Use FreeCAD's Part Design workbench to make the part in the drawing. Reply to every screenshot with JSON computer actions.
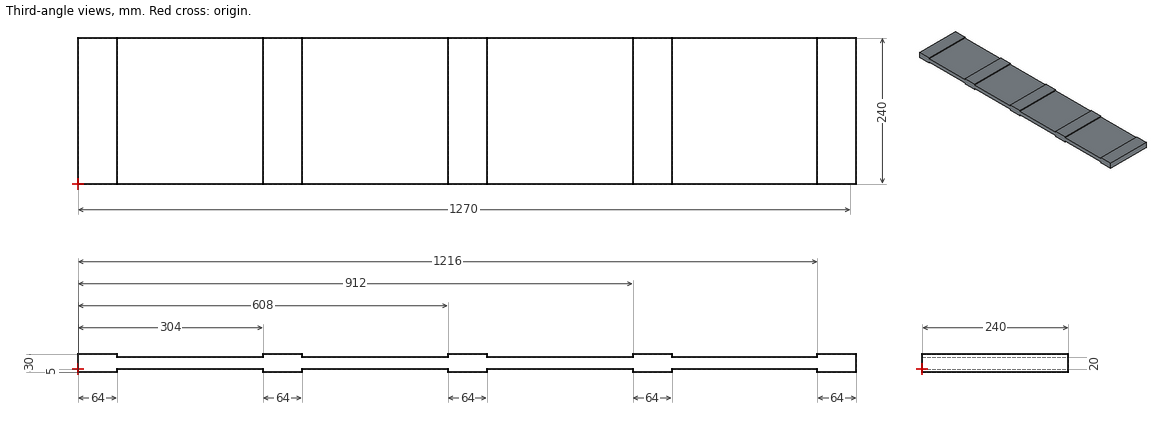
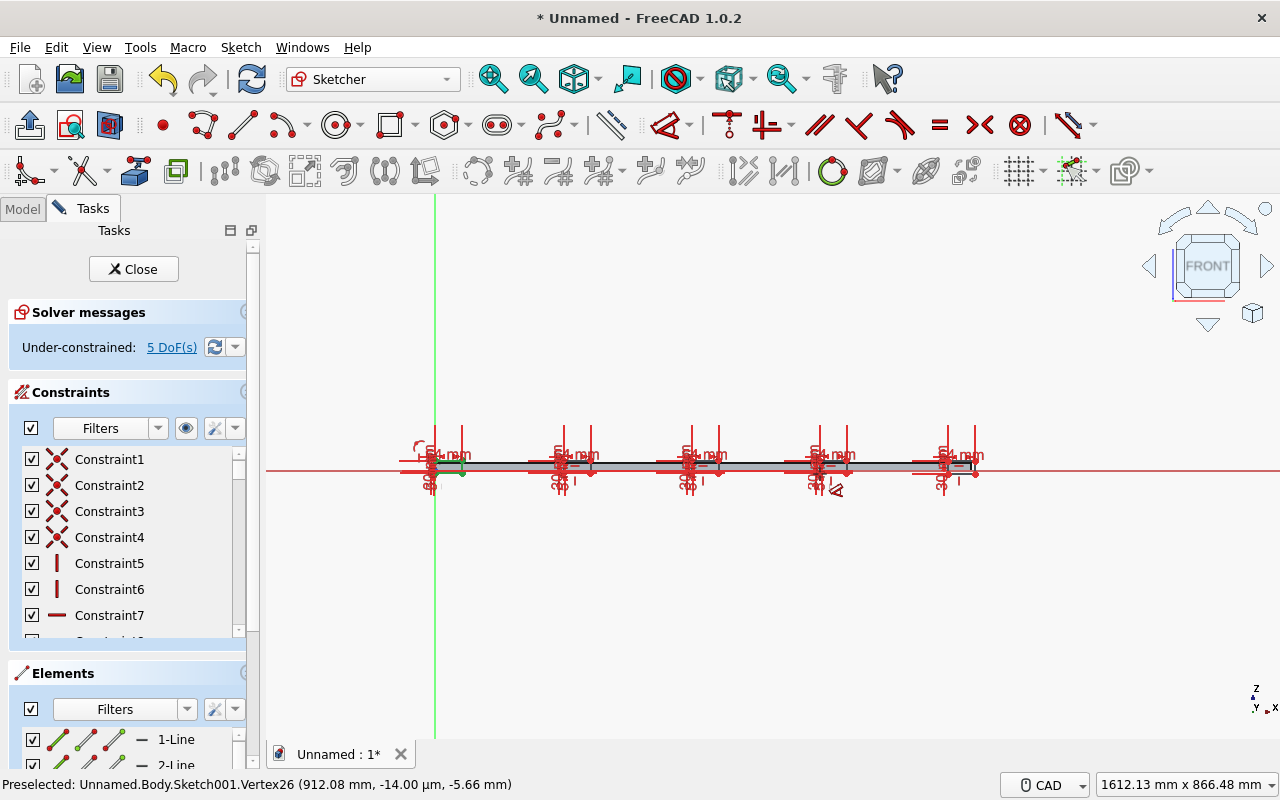
{"action": "scroll", "coordinate": [948, 474], "scroll_direction": "up", "scroll_amount": 15}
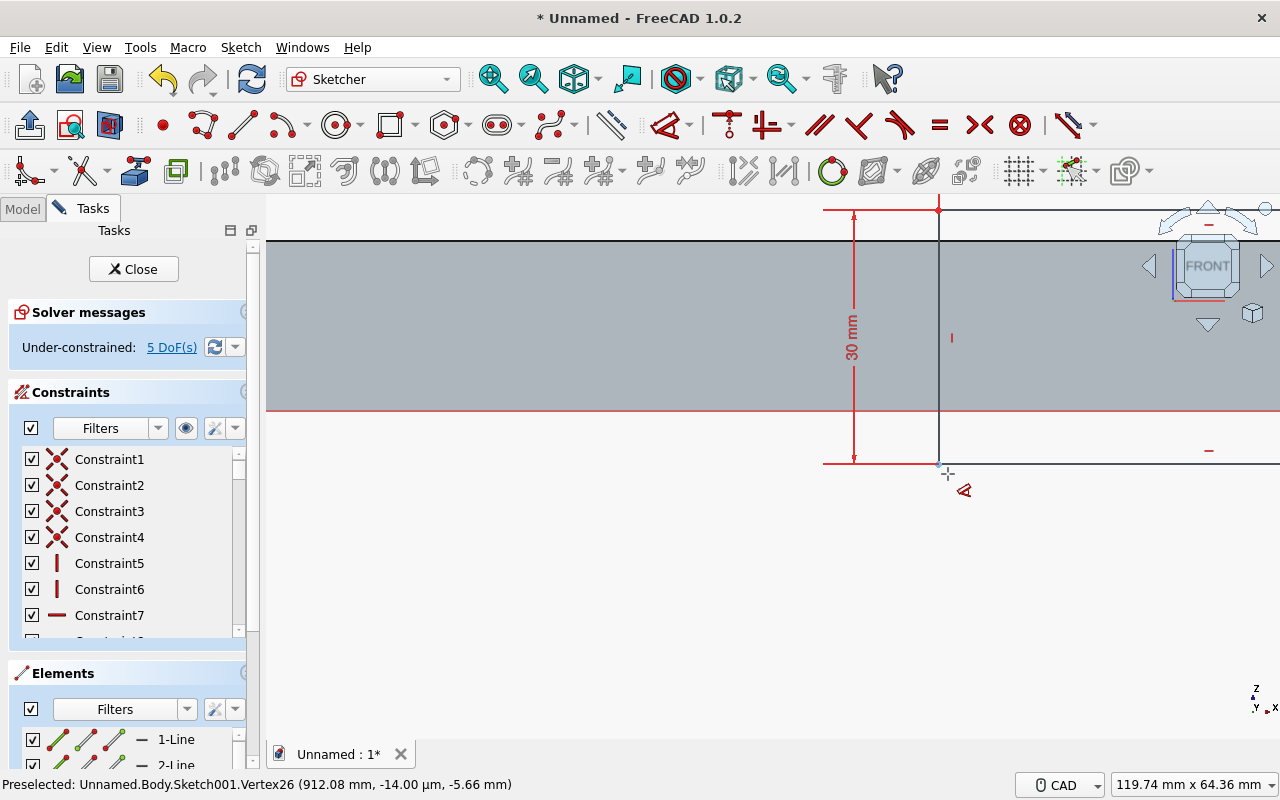
{"action": "left_click", "coordinate": [939, 464]}
{"action": "left_click", "coordinate": [973, 438]}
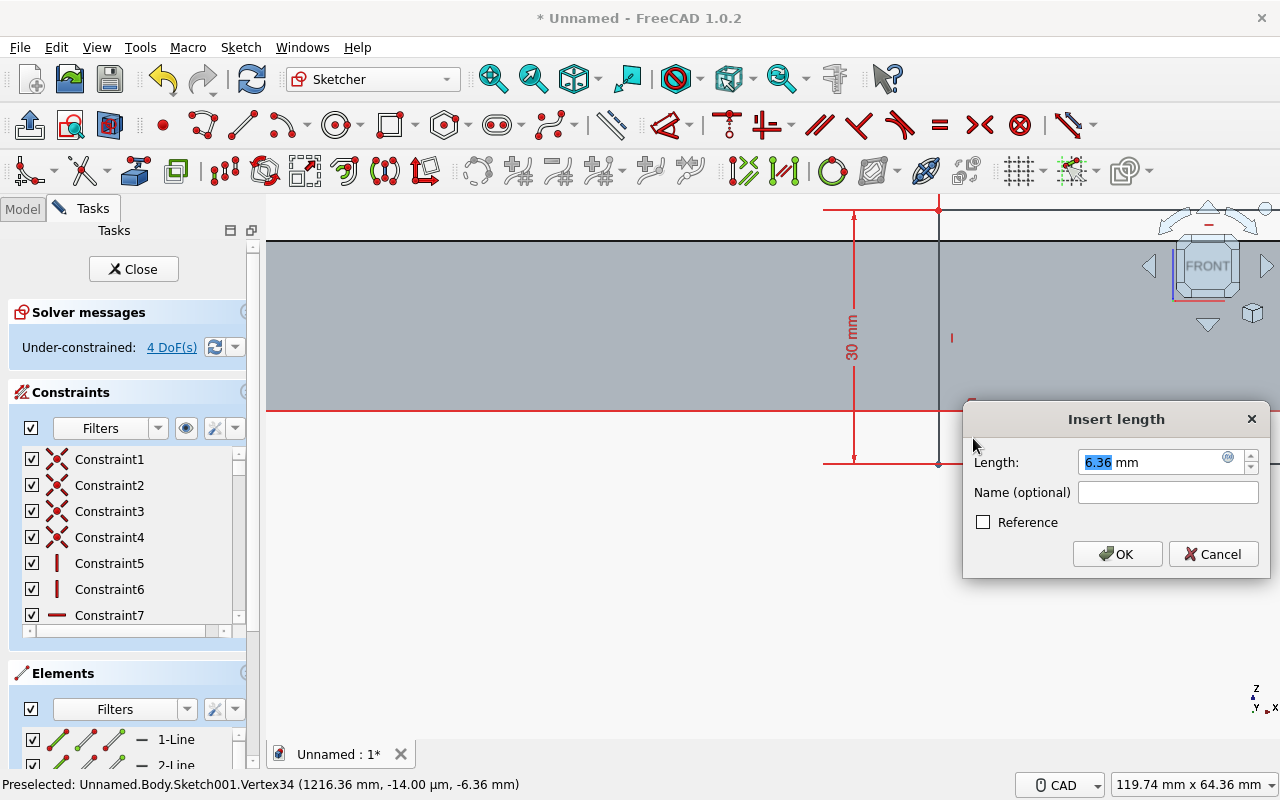
{"action": "type", "text": "5"}
{"action": "key", "text": "Return"}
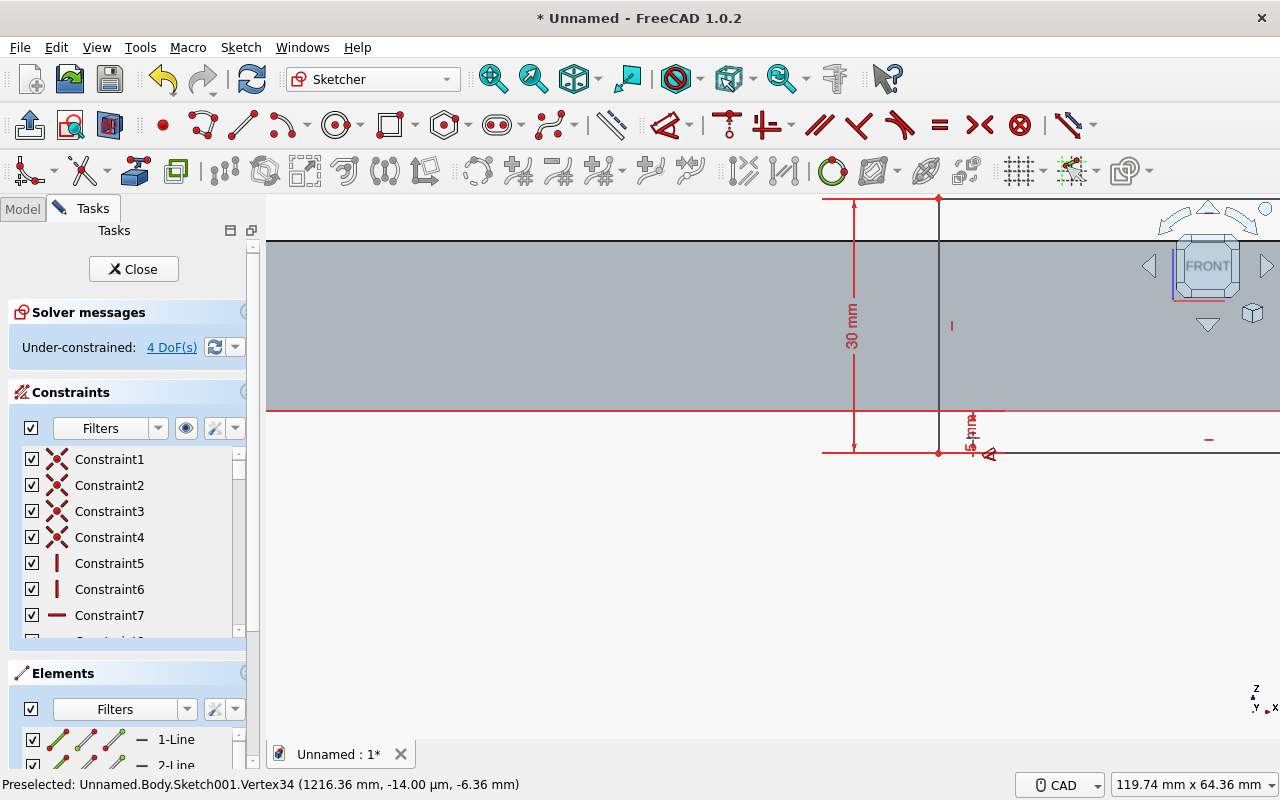
{"action": "scroll", "coordinate": [948, 474], "scroll_direction": "down", "scroll_amount": 15}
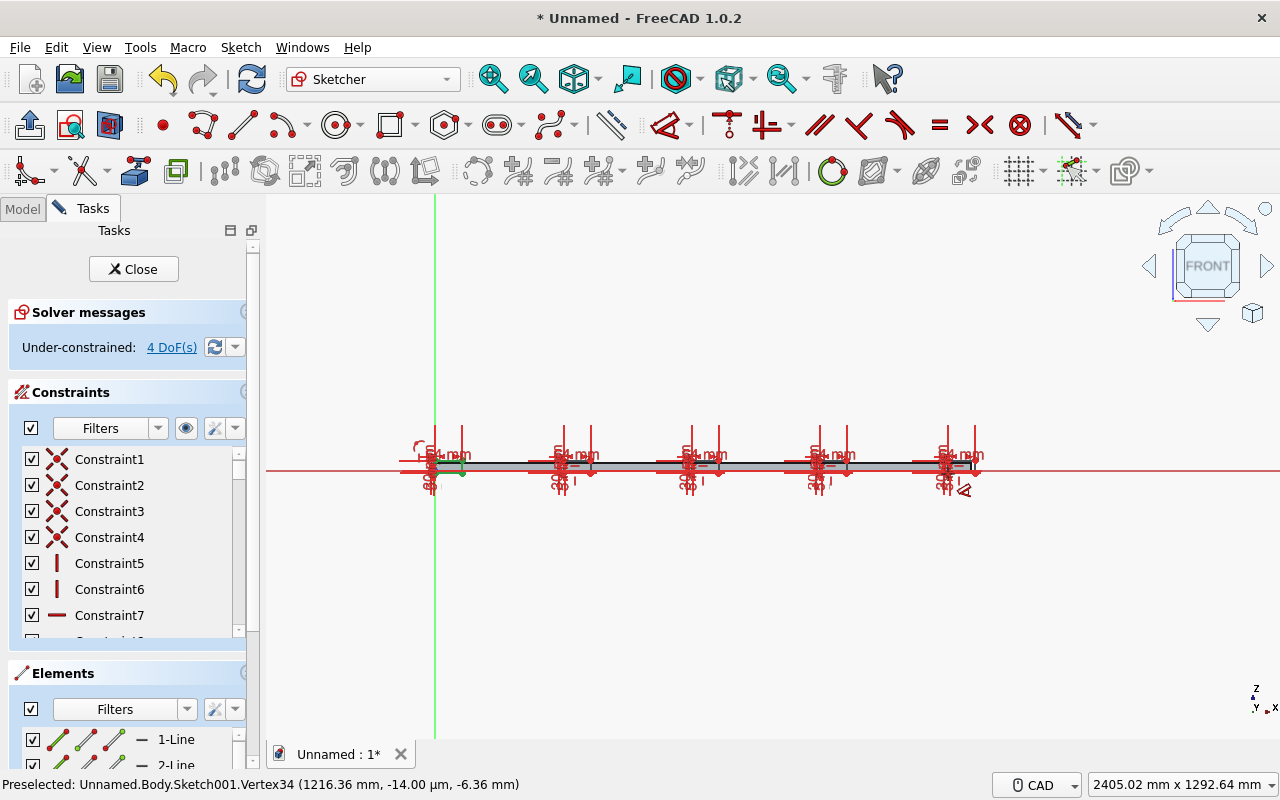
{"action": "left_click", "coordinate": [564, 461]}
{"action": "left_click", "coordinate": [499, 427]}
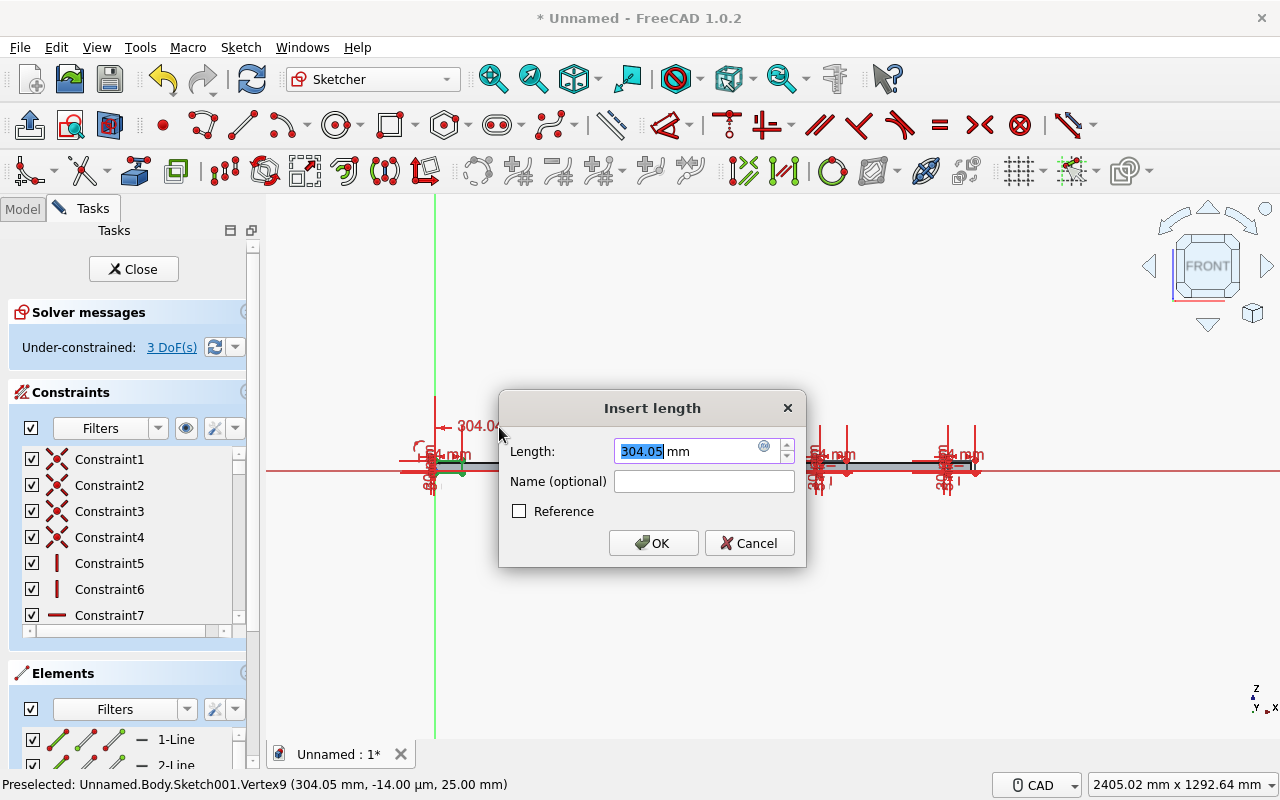
{"action": "type", "text": "304"}
{"action": "key", "text": "Return"}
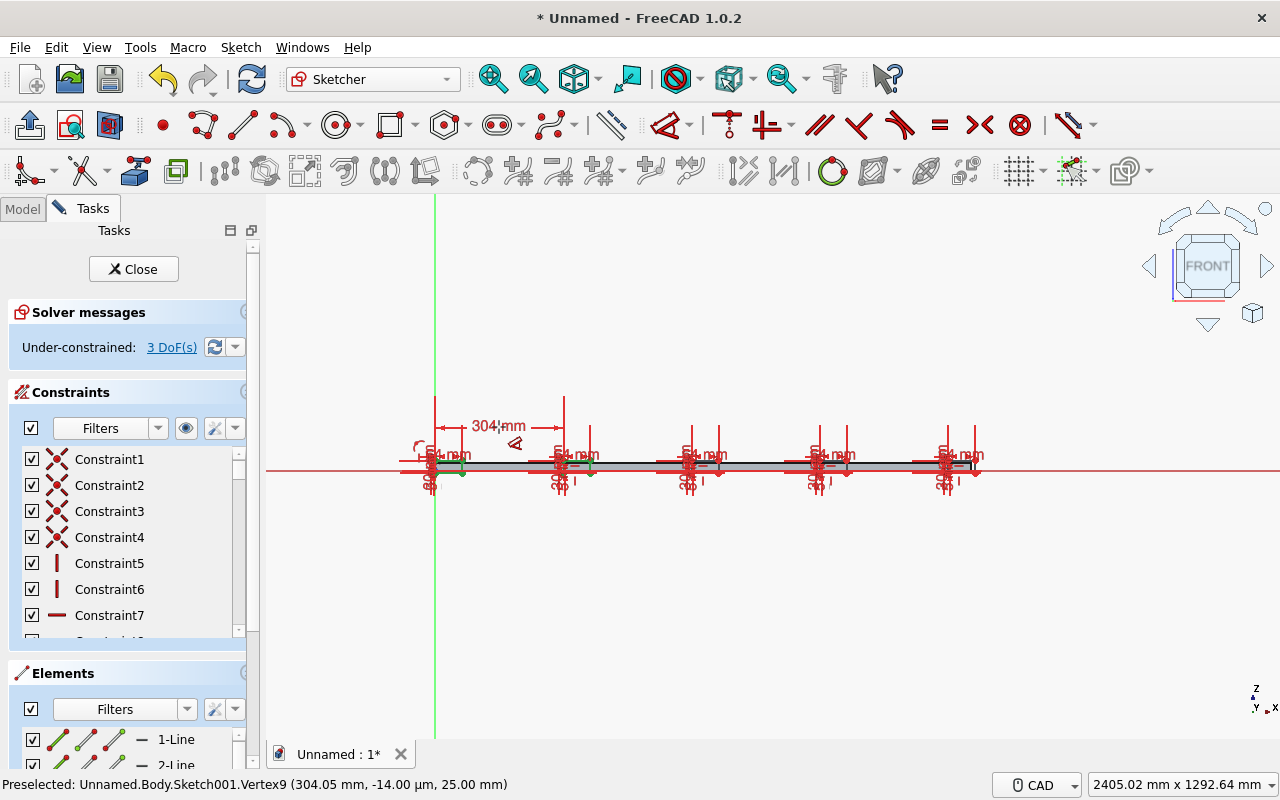
{"action": "left_click", "coordinate": [692, 461]}
{"action": "left_click", "coordinate": [622, 427]}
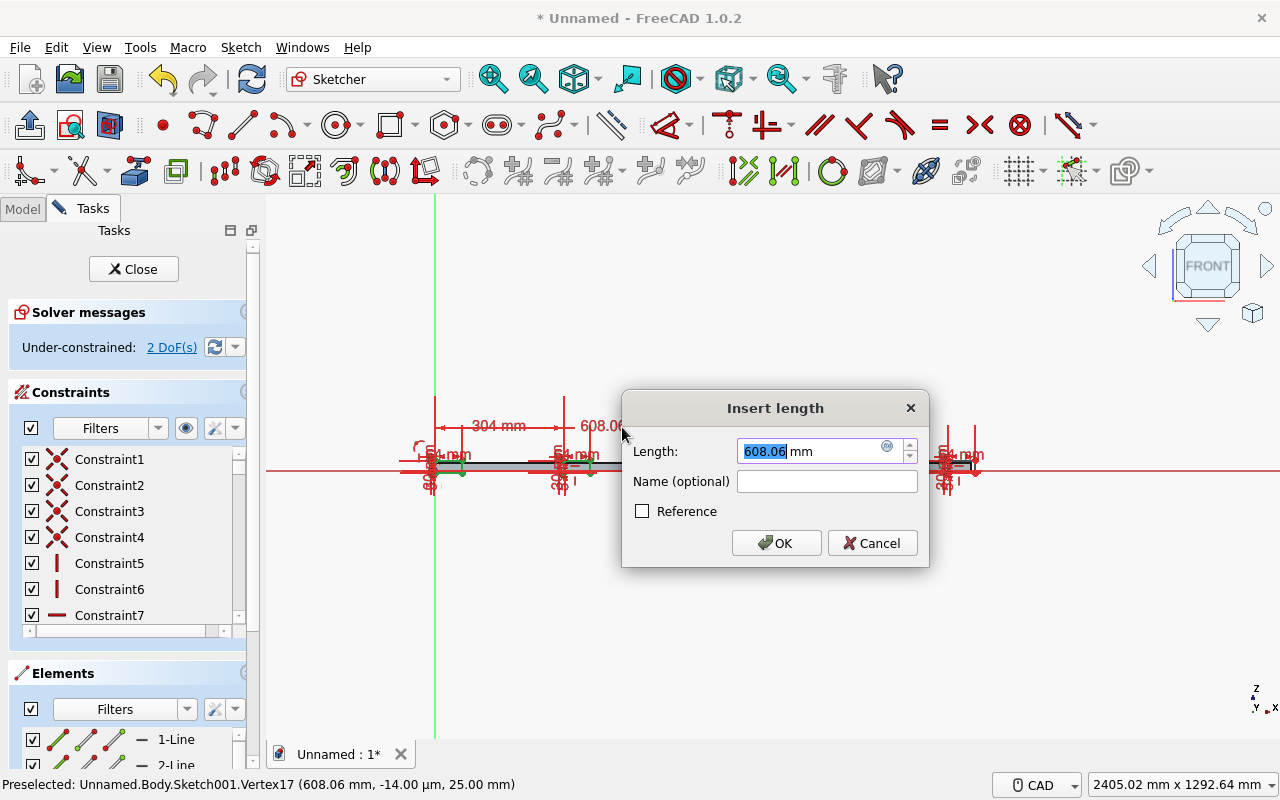
{"action": "type", "text": "608"}
{"action": "key", "text": "Return"}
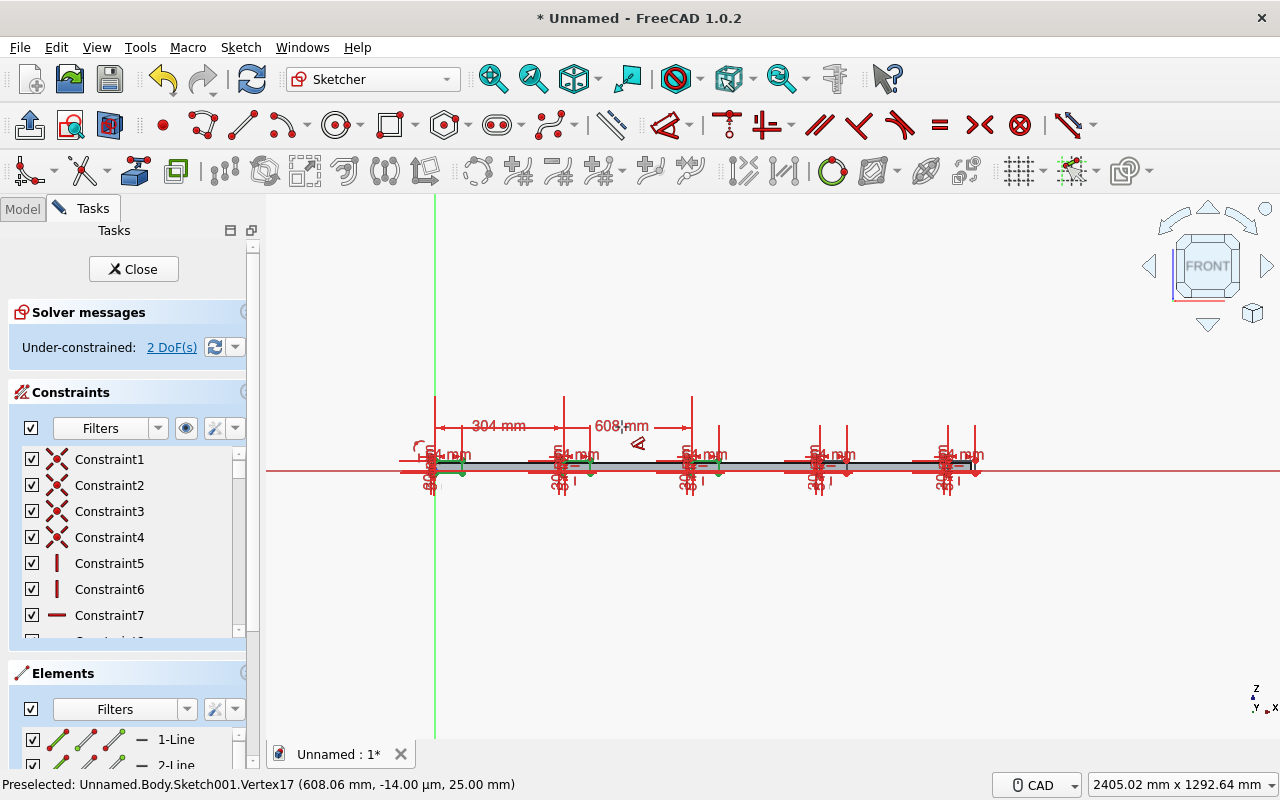
{"action": "left_click", "coordinate": [820, 461]}
{"action": "left_click", "coordinate": [716, 427]}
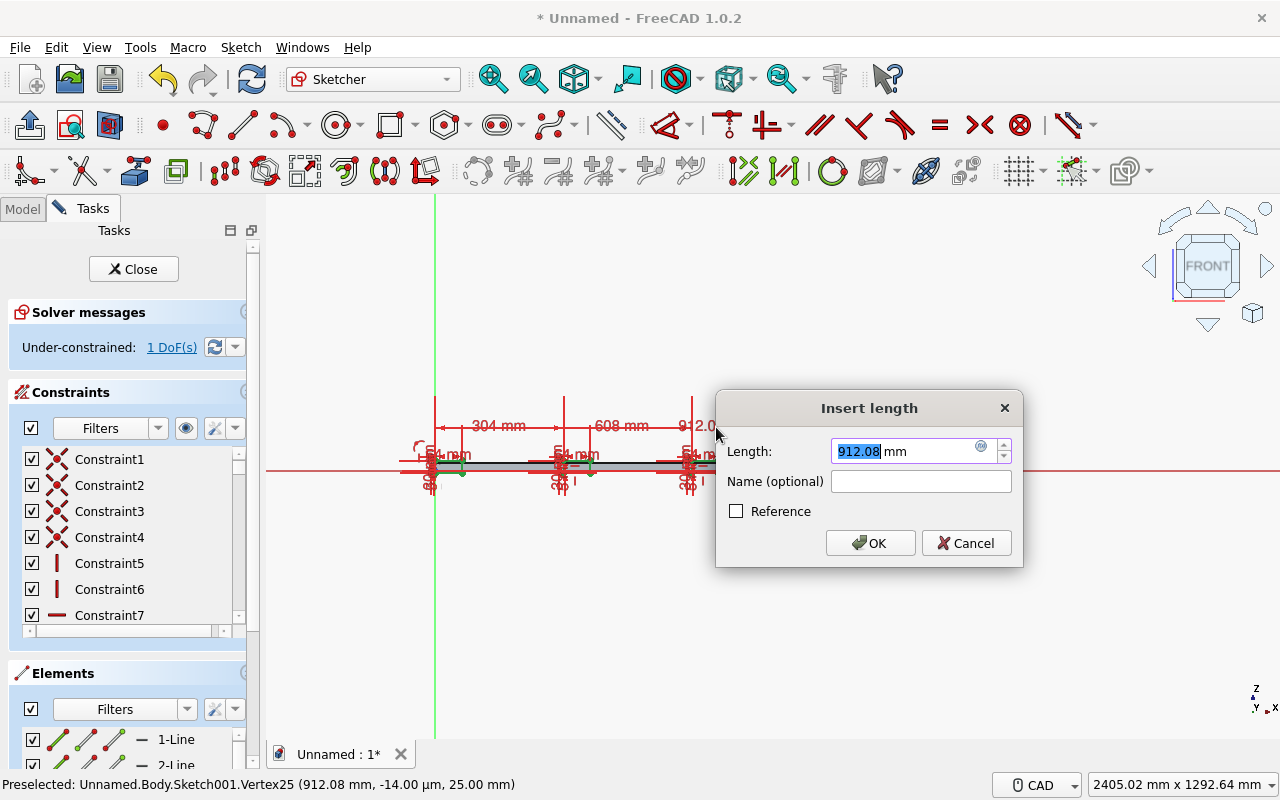
{"action": "type", "text": "912"}
{"action": "key", "text": "Return"}